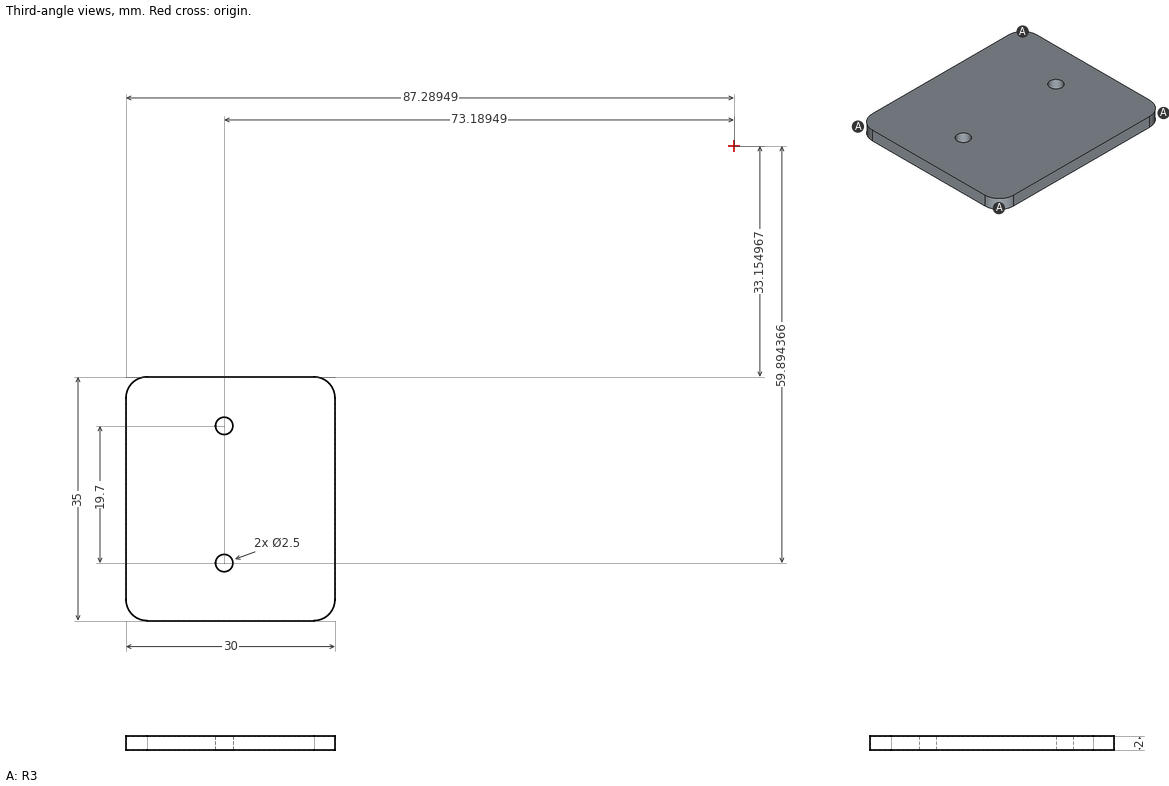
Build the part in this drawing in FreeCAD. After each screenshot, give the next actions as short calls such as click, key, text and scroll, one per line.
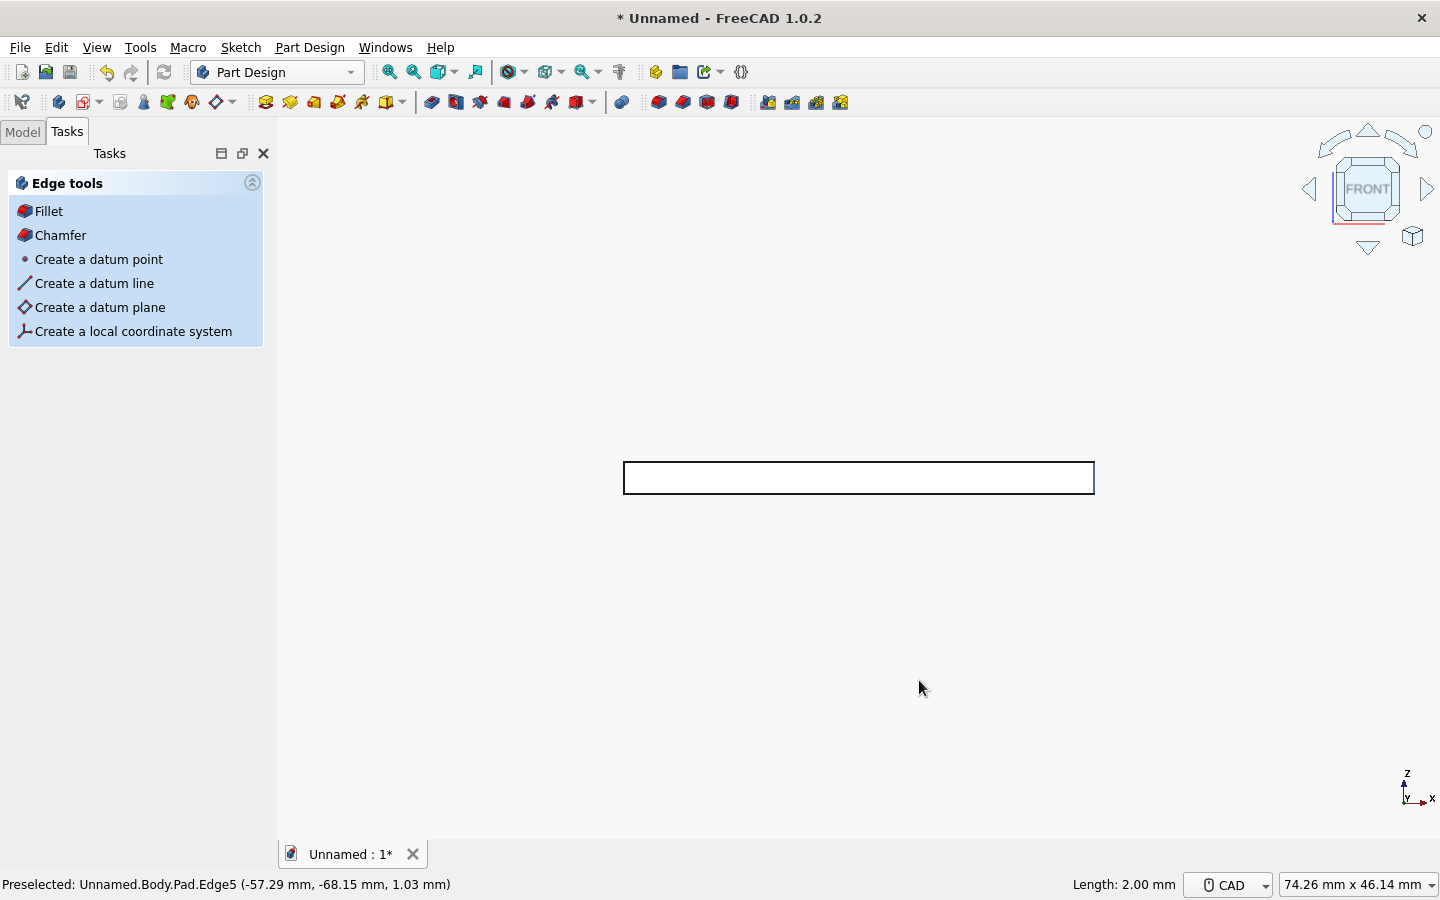
click(390, 72)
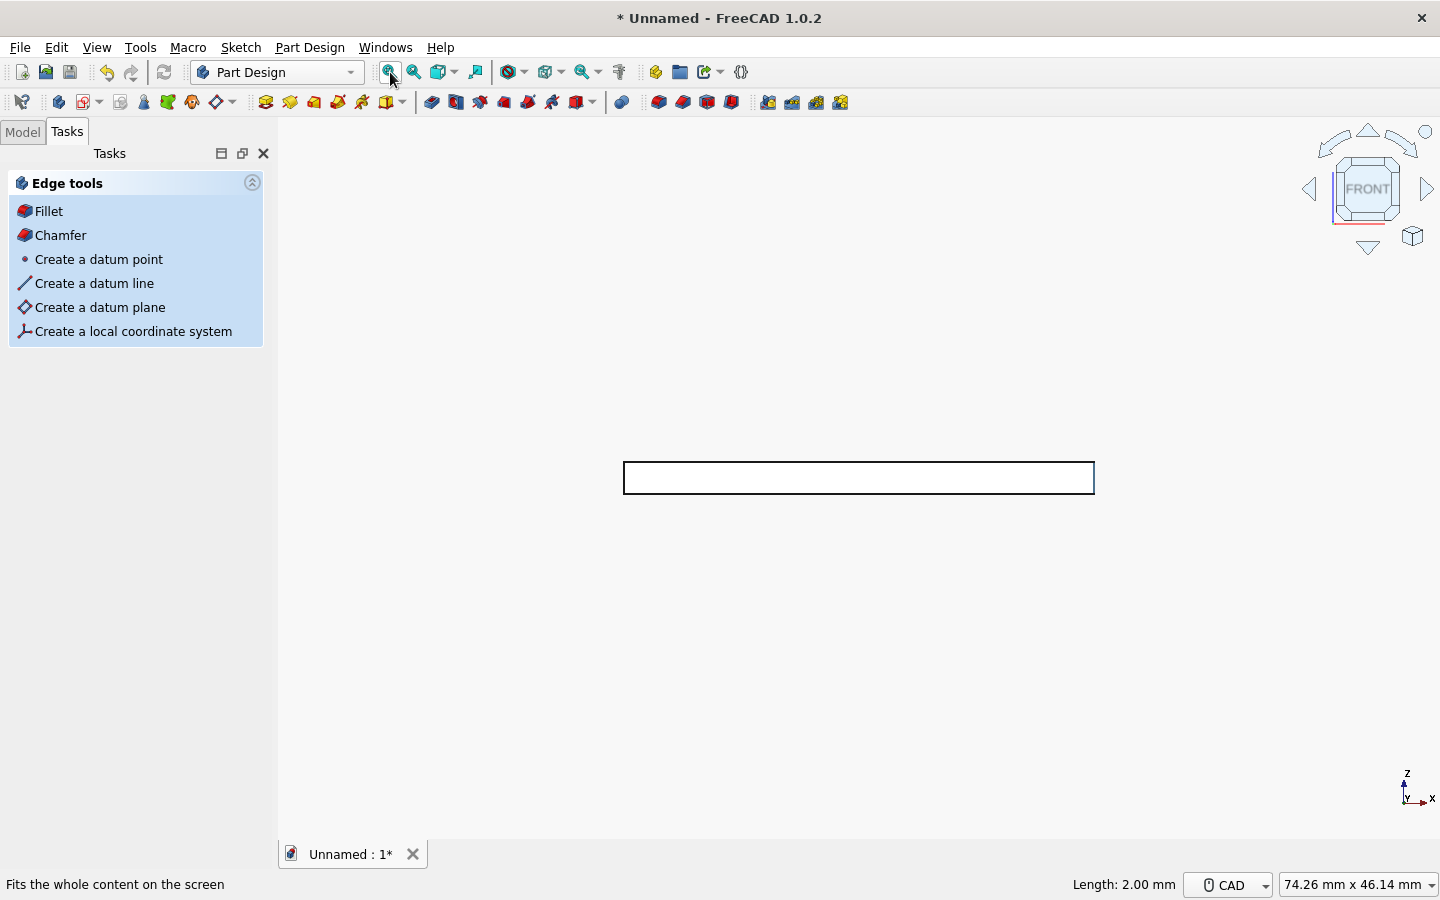
click(624, 477, ctrl)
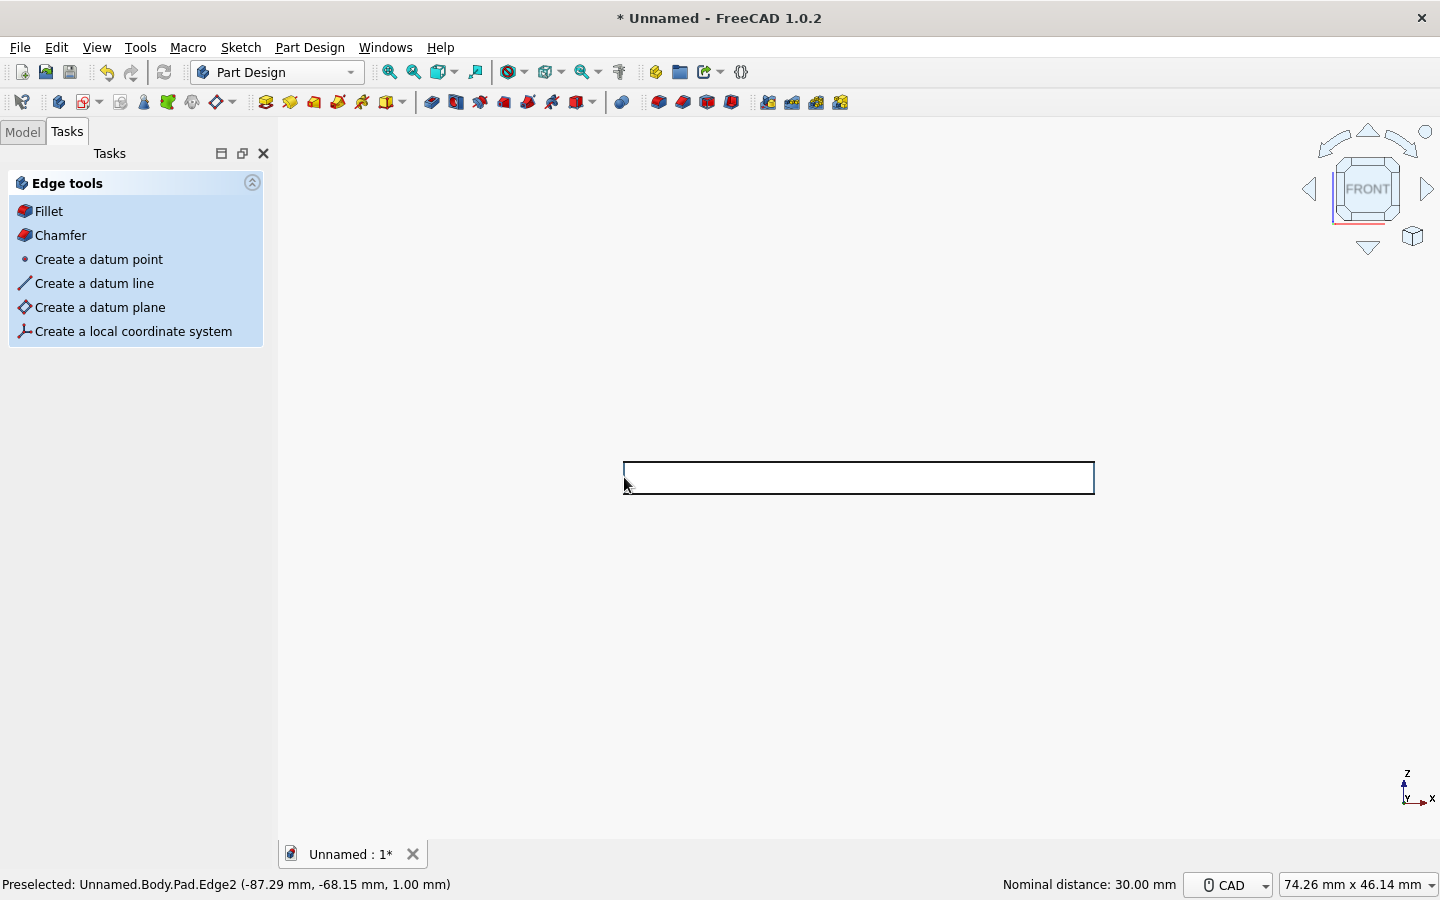
key(3)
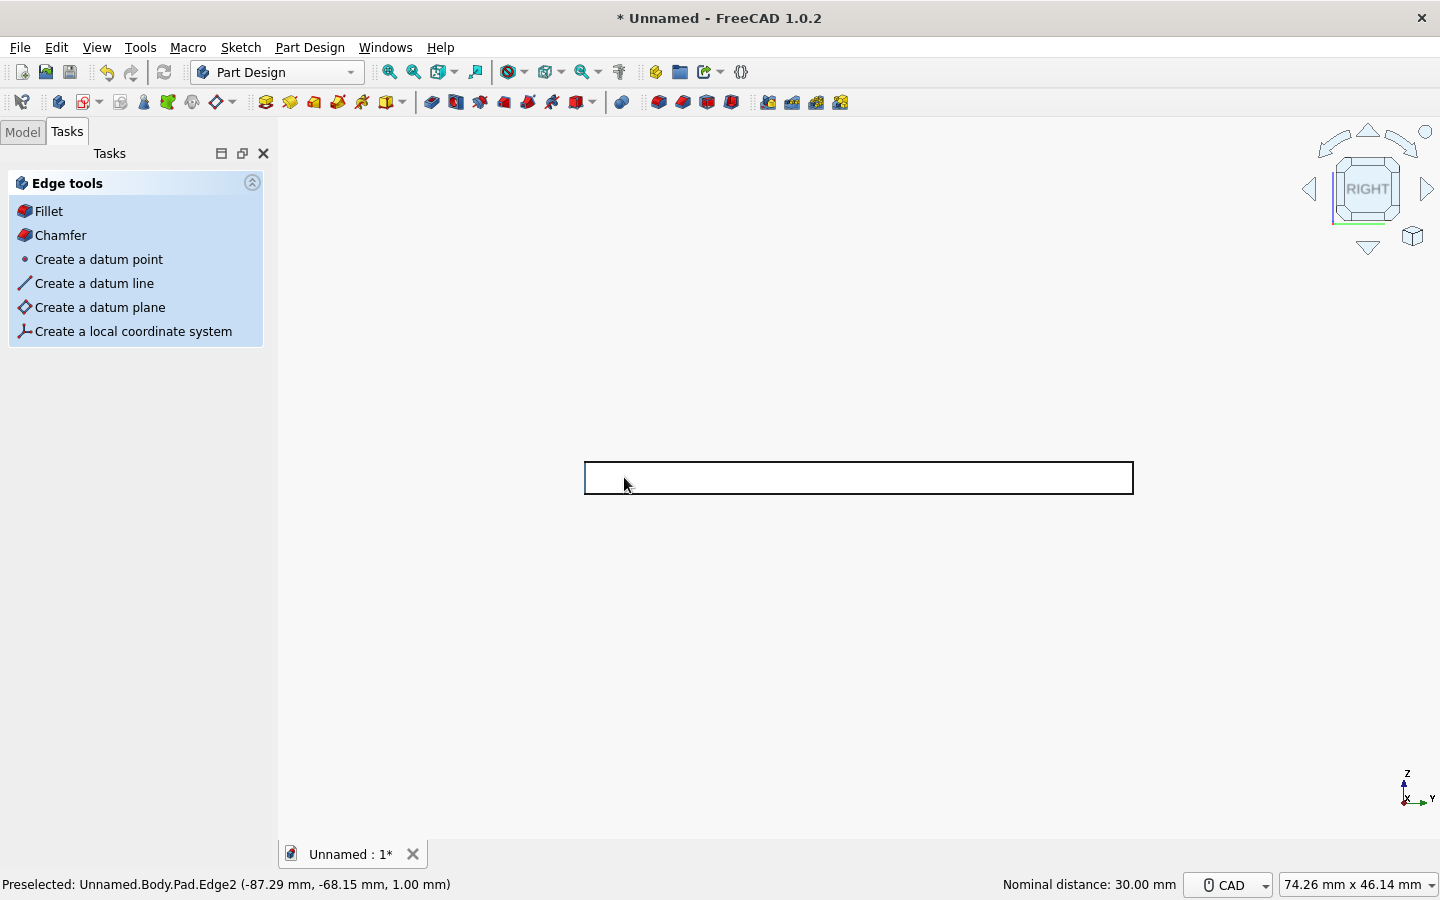
click(1133, 477, ctrl)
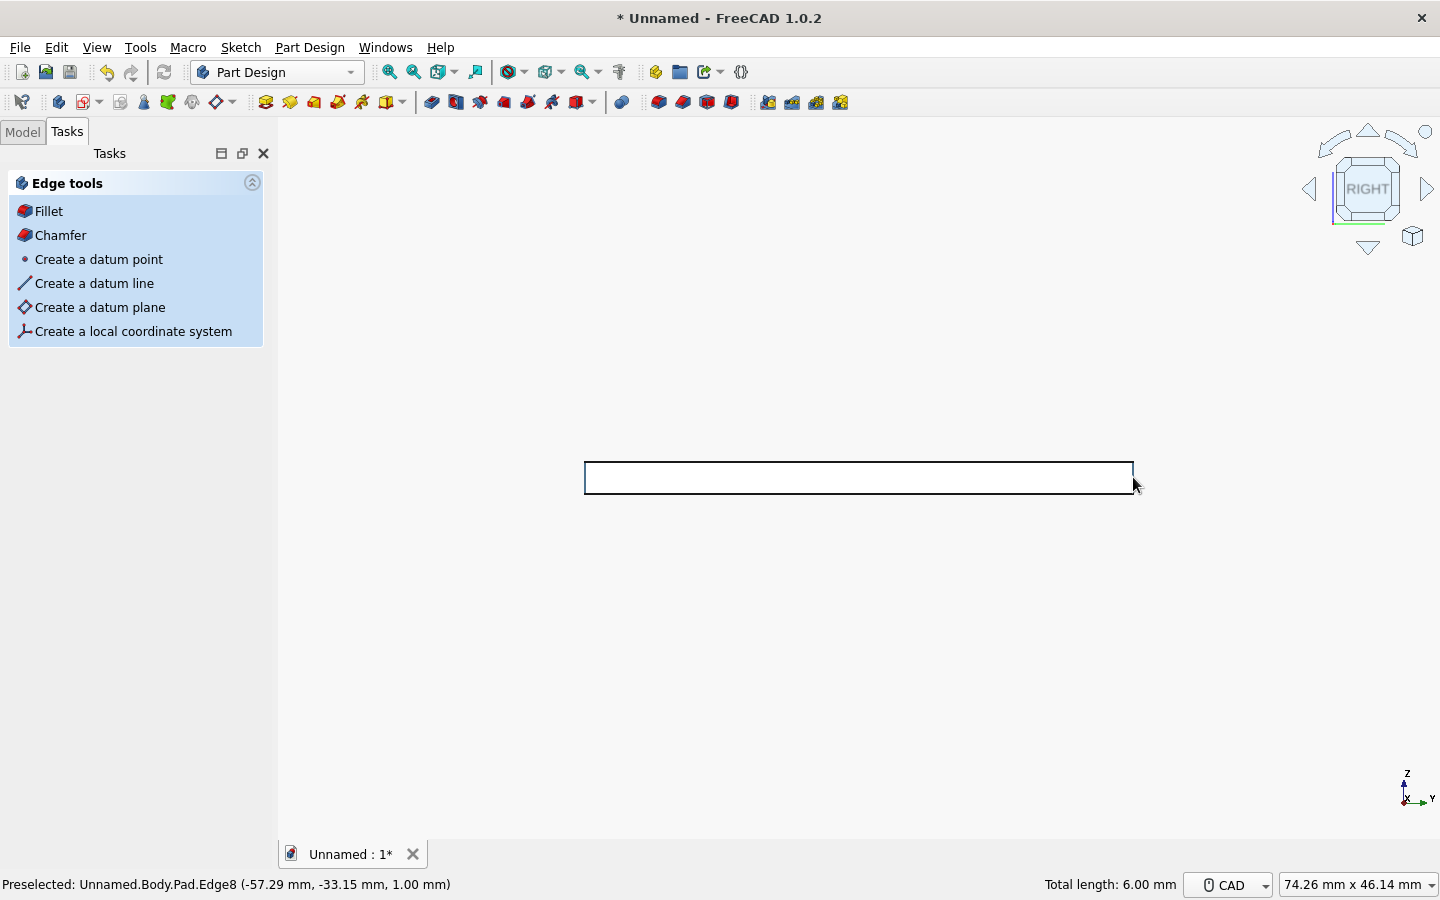
key(5)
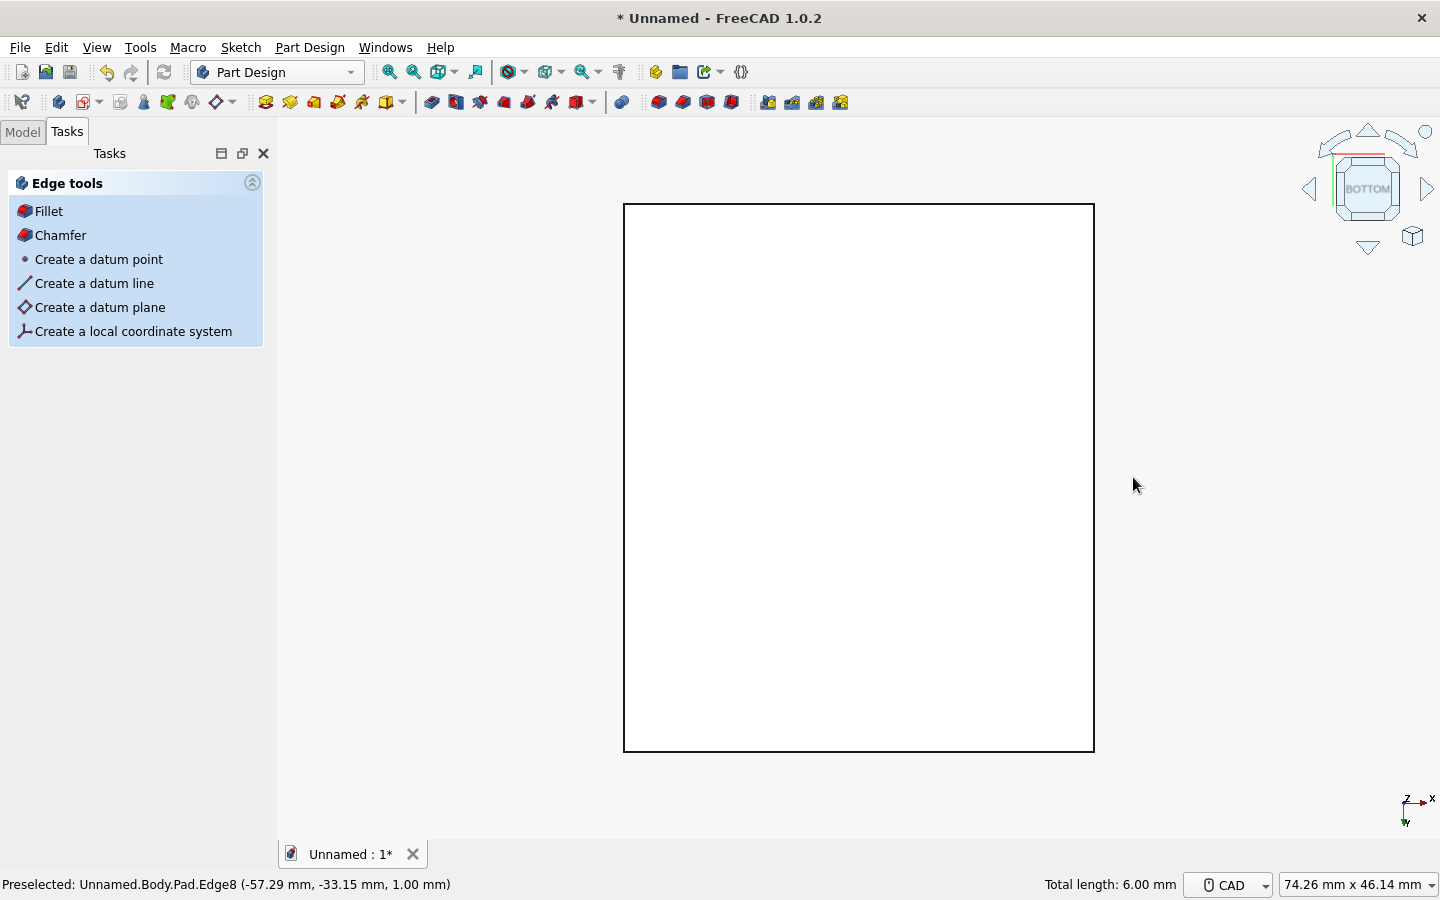
key(4)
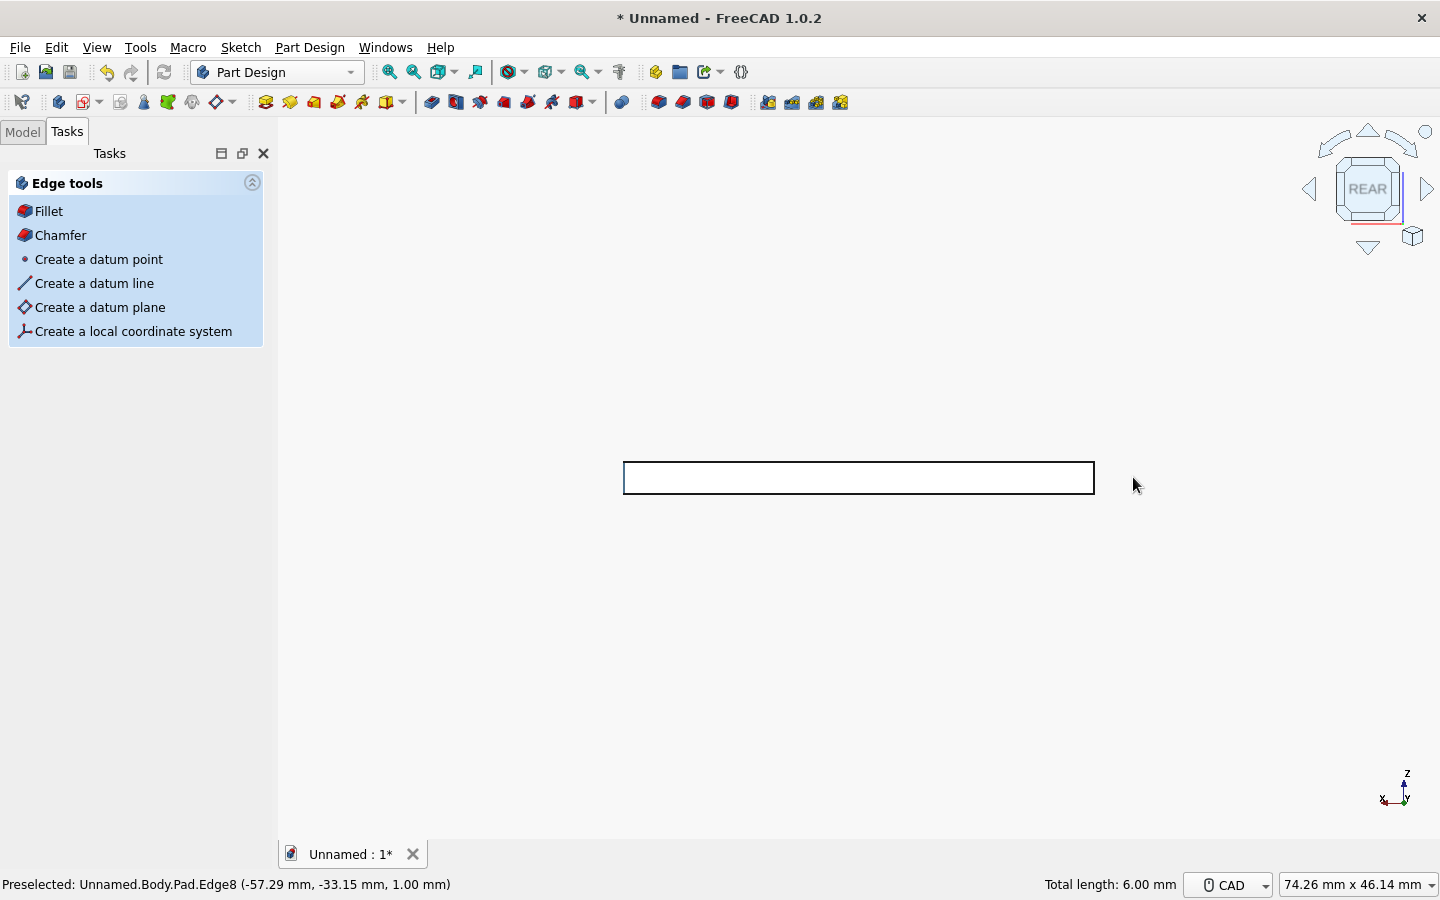
key(v)
key(f)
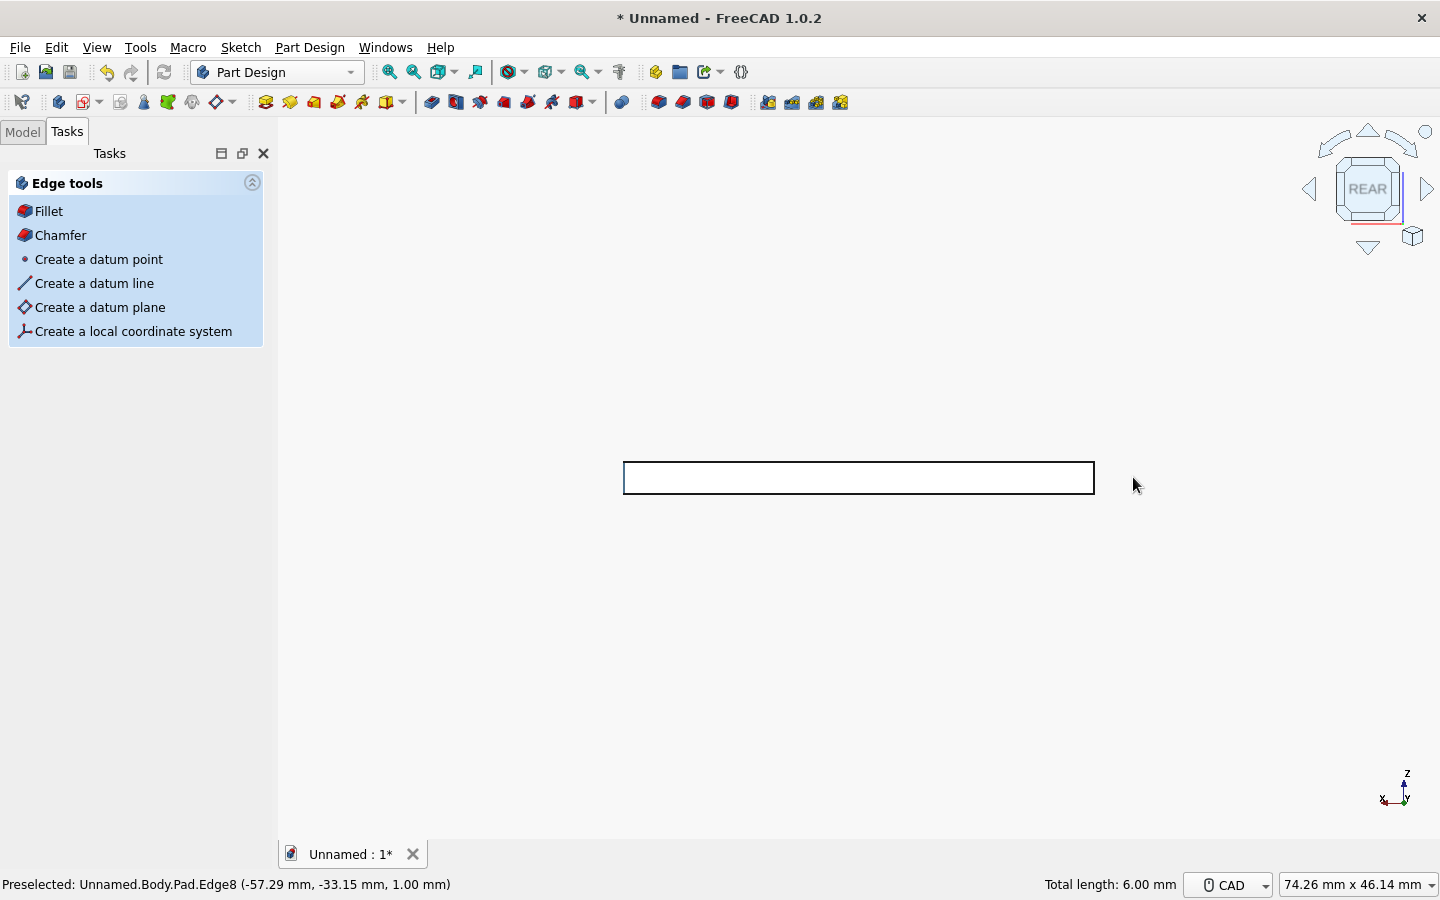
click(1094, 477, ctrl)